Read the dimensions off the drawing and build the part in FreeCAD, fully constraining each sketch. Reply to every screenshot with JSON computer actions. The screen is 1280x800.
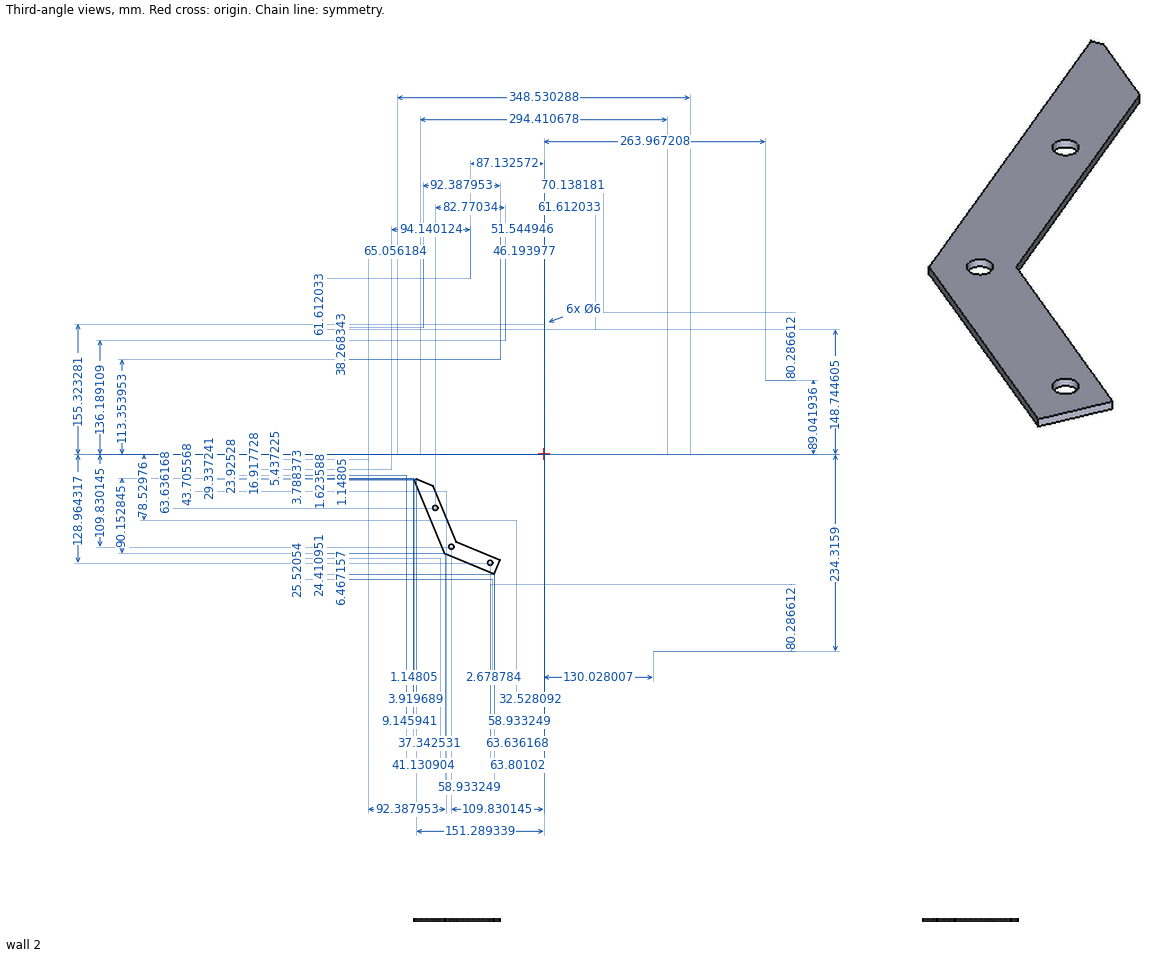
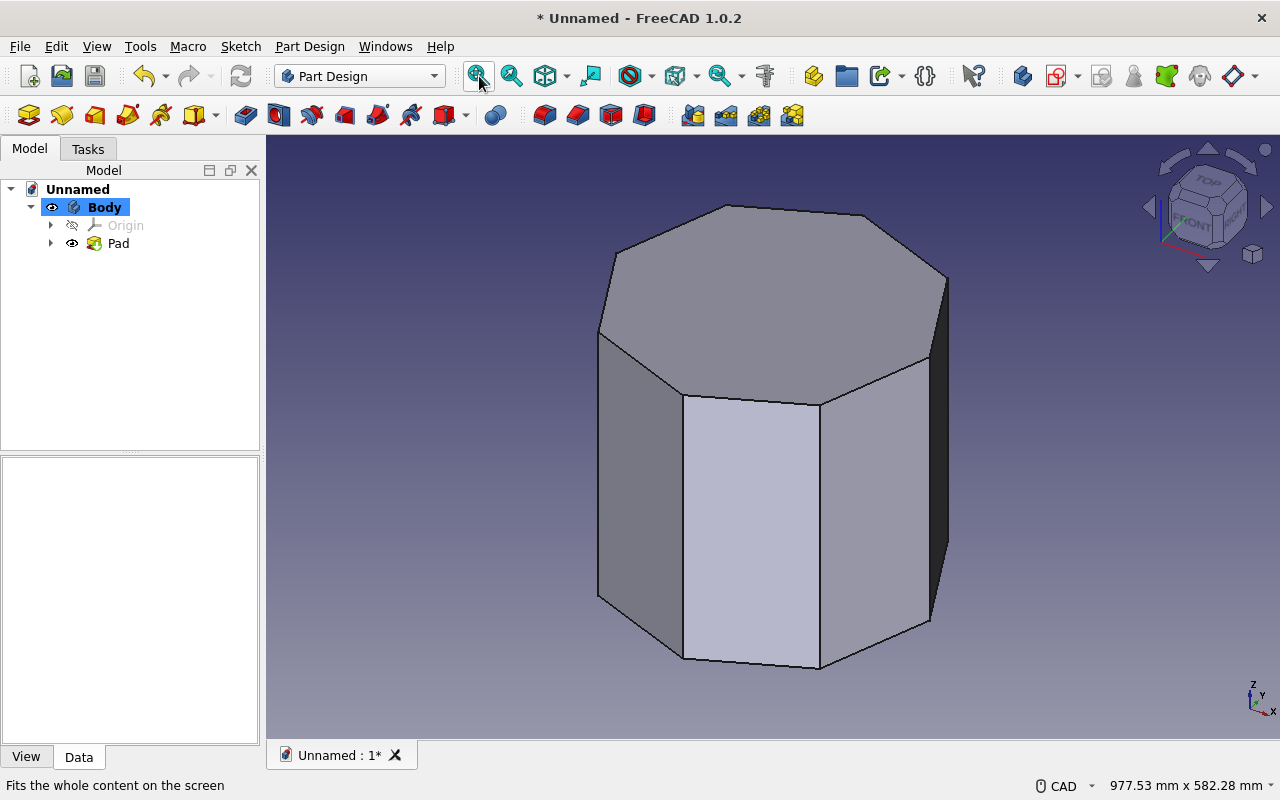
{"action": "key", "text": "0"}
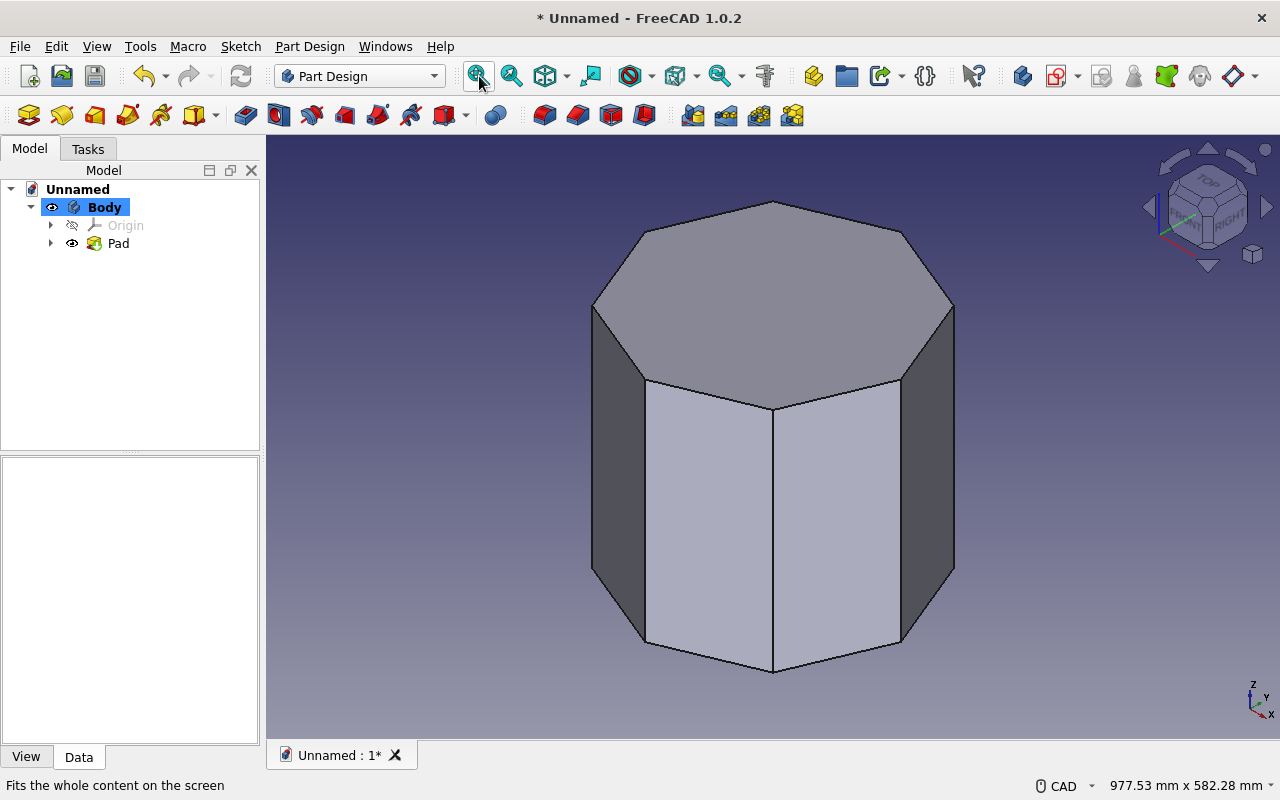
{"action": "key", "text": "2"}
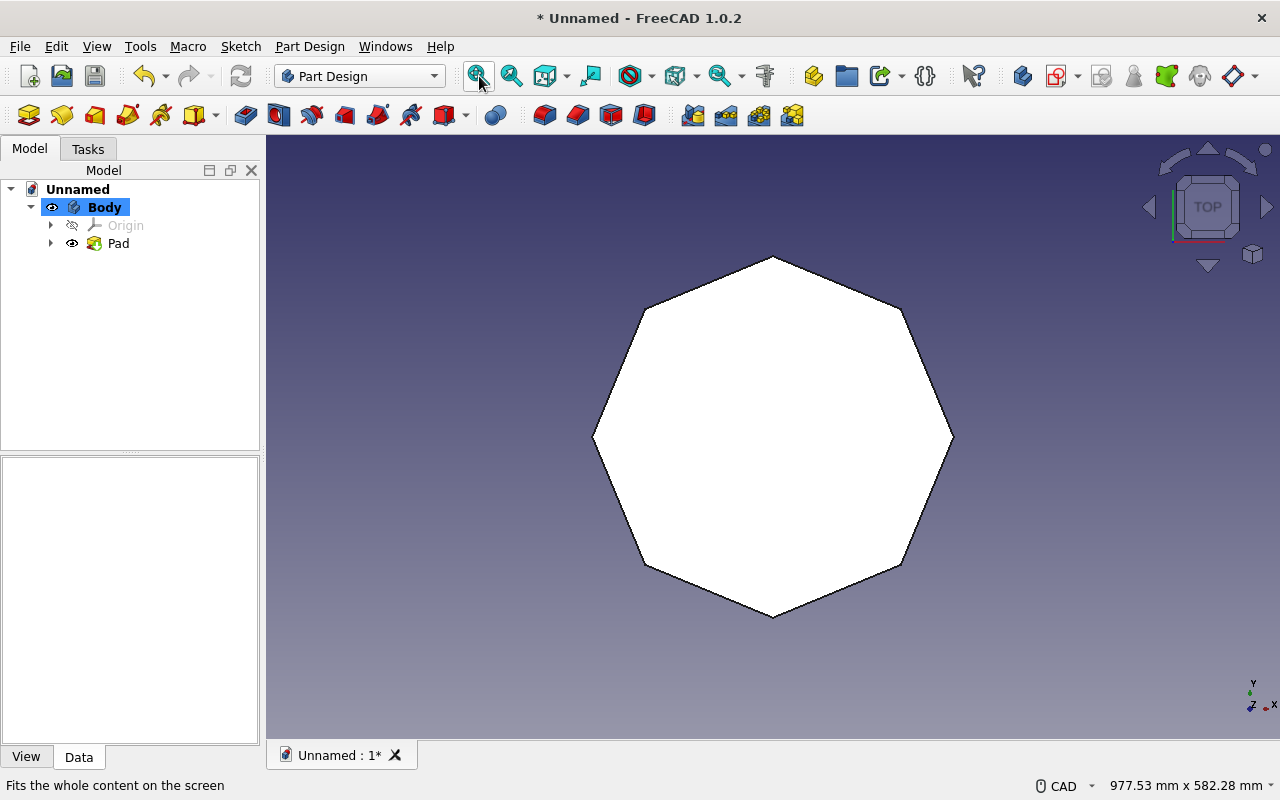
{"action": "key", "text": "1"}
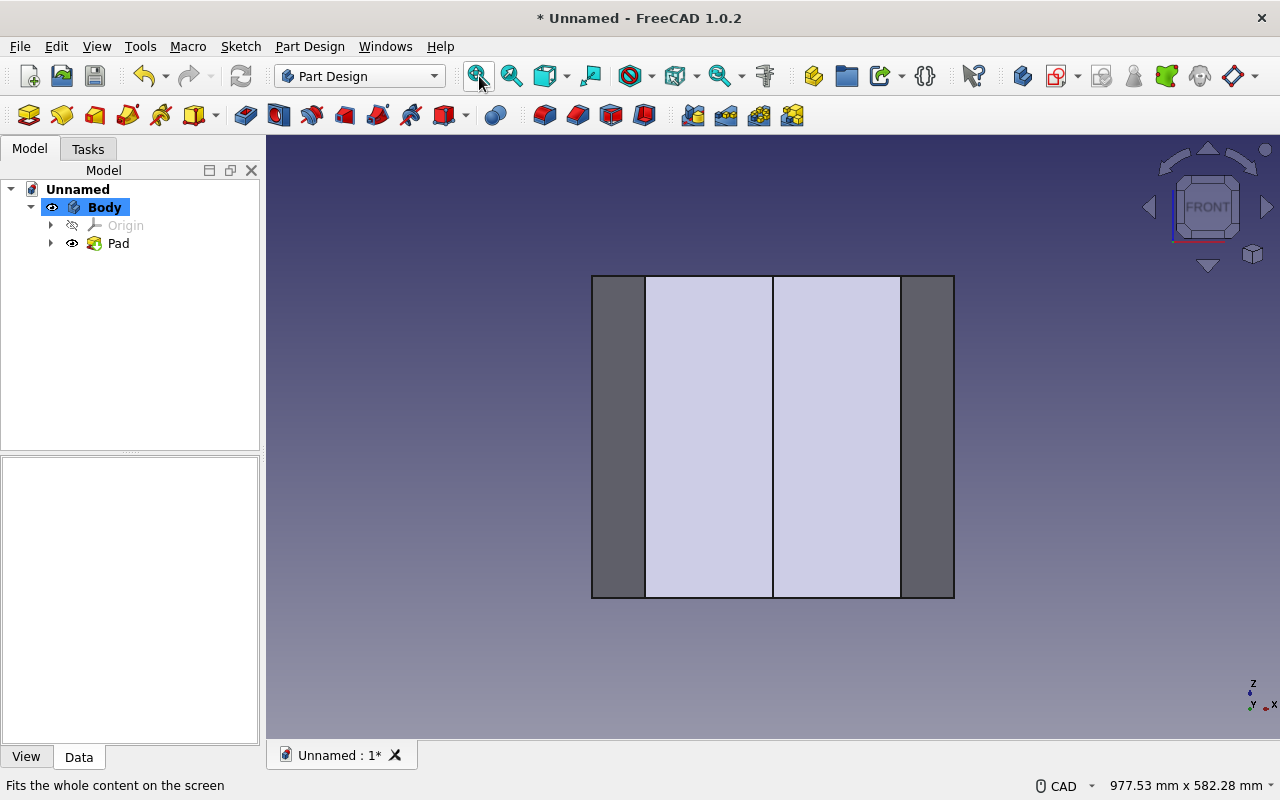
{"action": "key", "text": "3"}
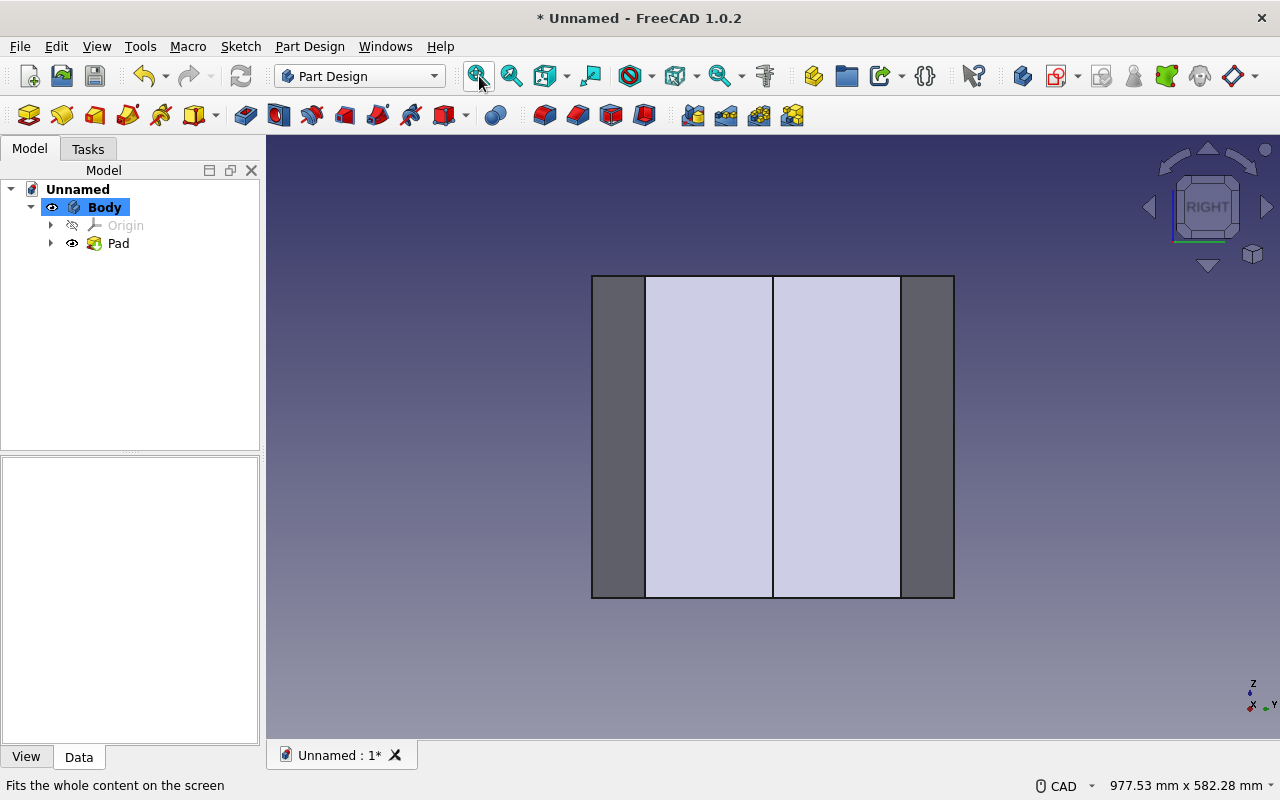
{"action": "key", "text": "5"}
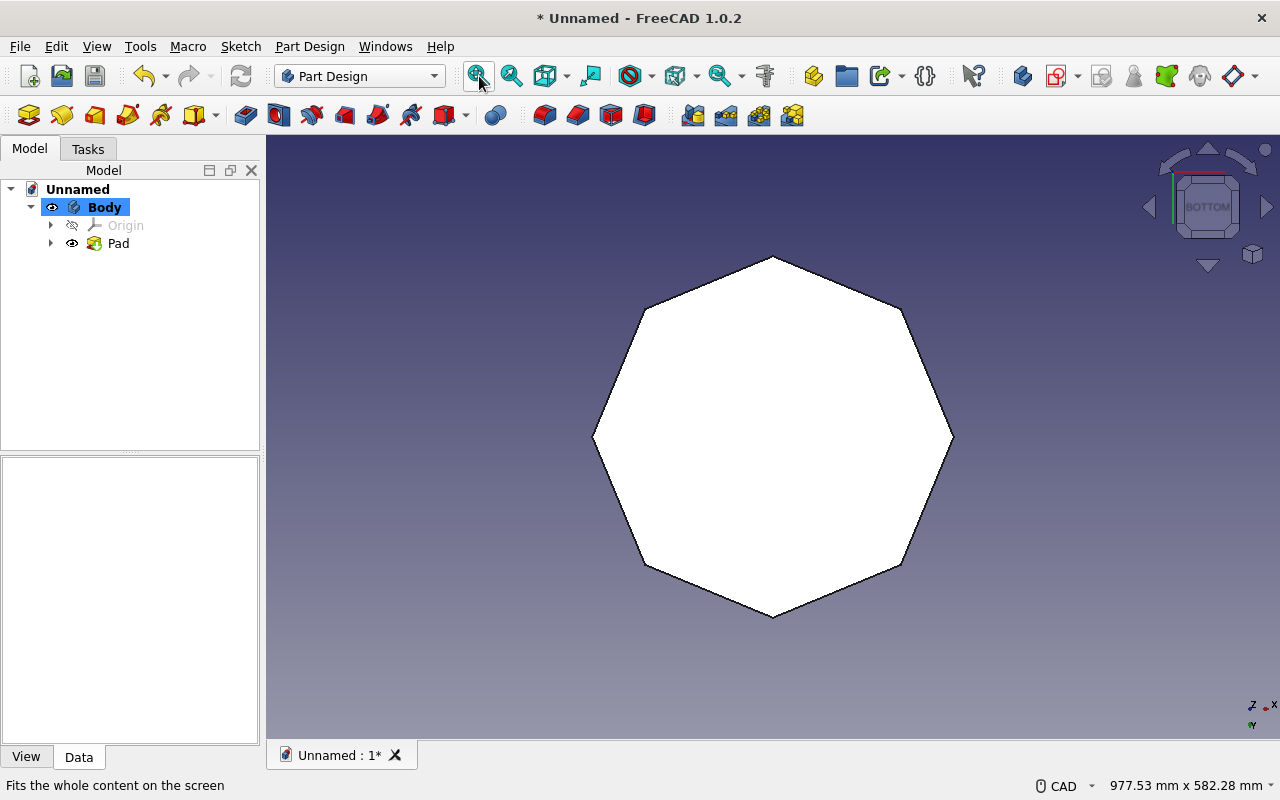
{"action": "left_click", "coordinate": [773, 436]}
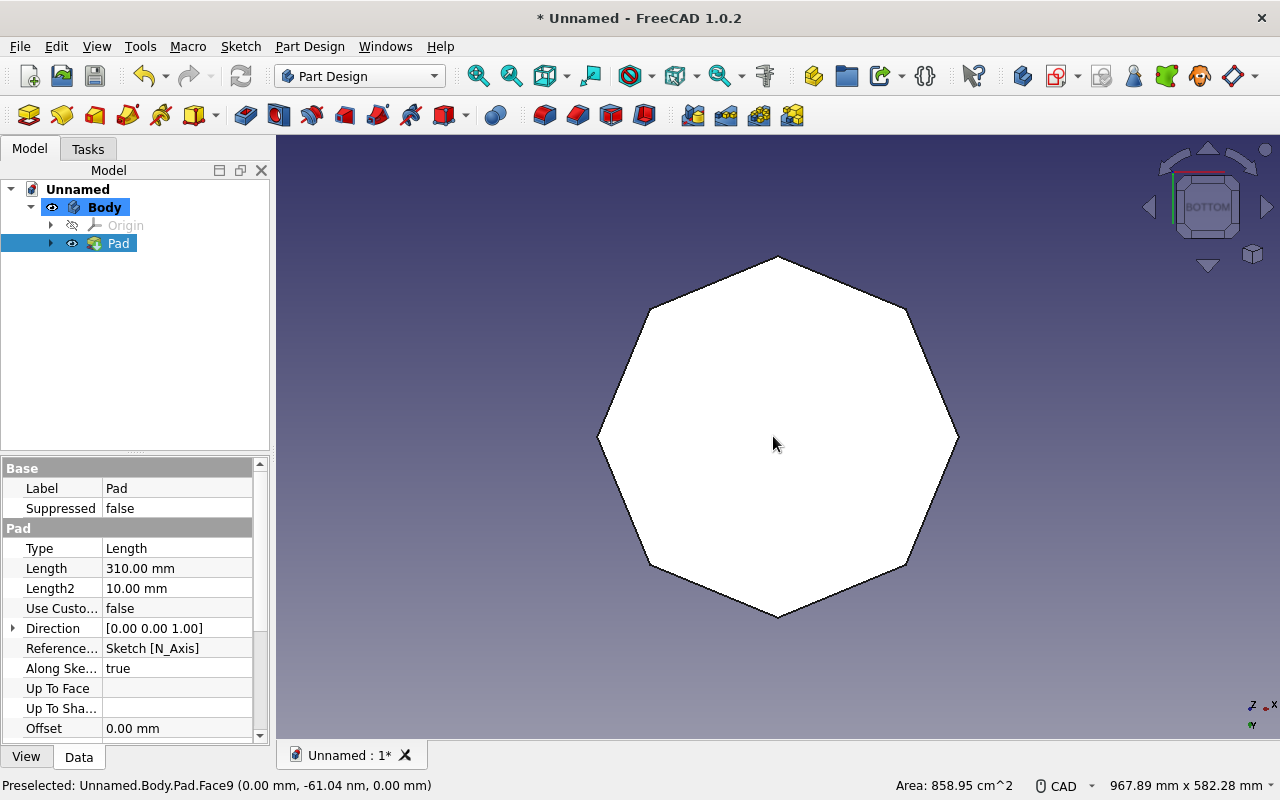
{"action": "left_click", "coordinate": [644, 116]}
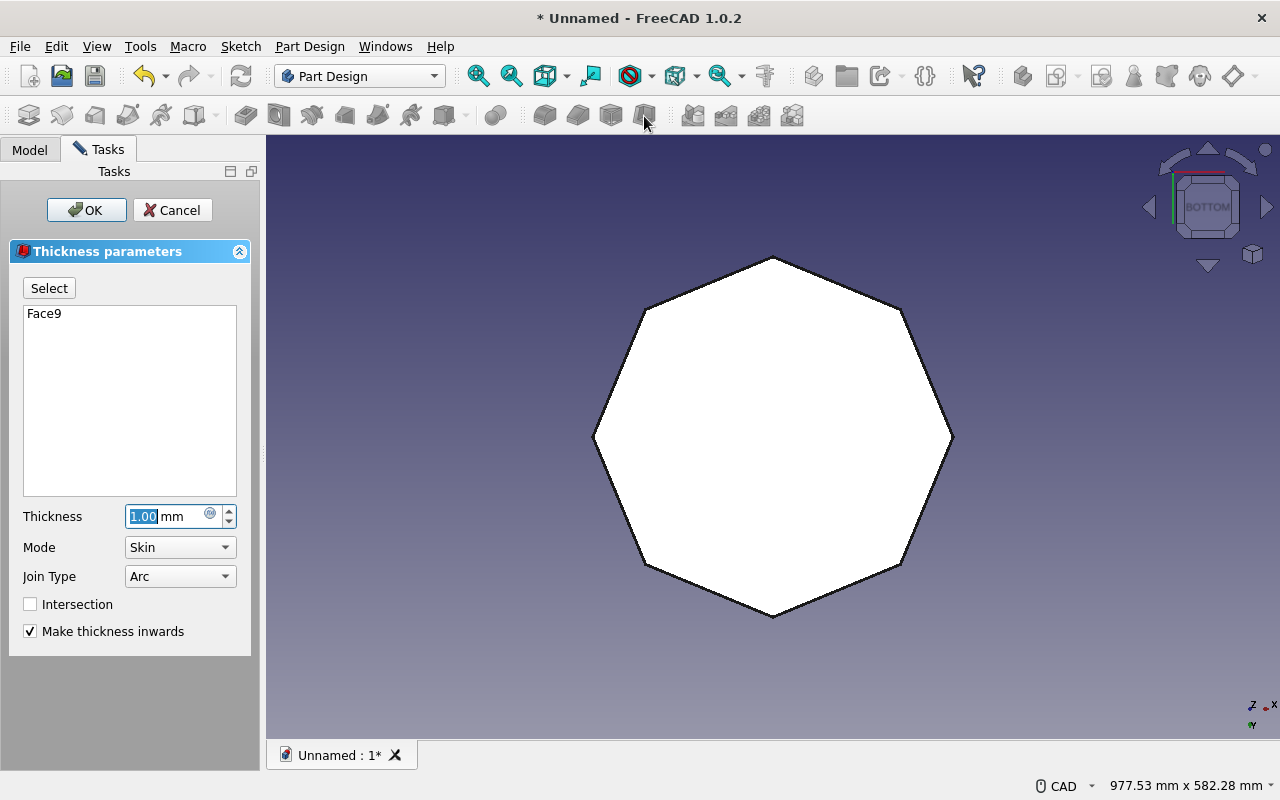
{"action": "type", "text": "2"}
{"action": "key", "text": "Tab"}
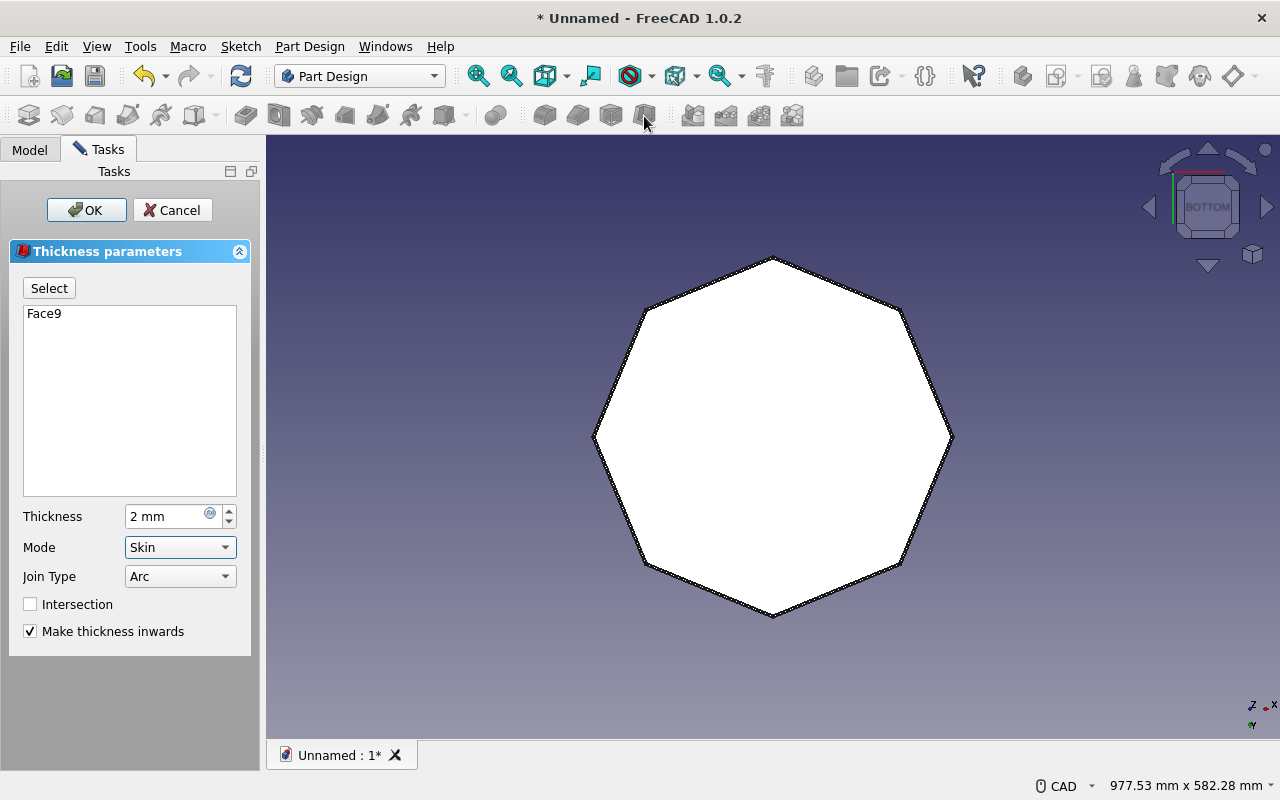
{"action": "left_click", "coordinate": [181, 576]}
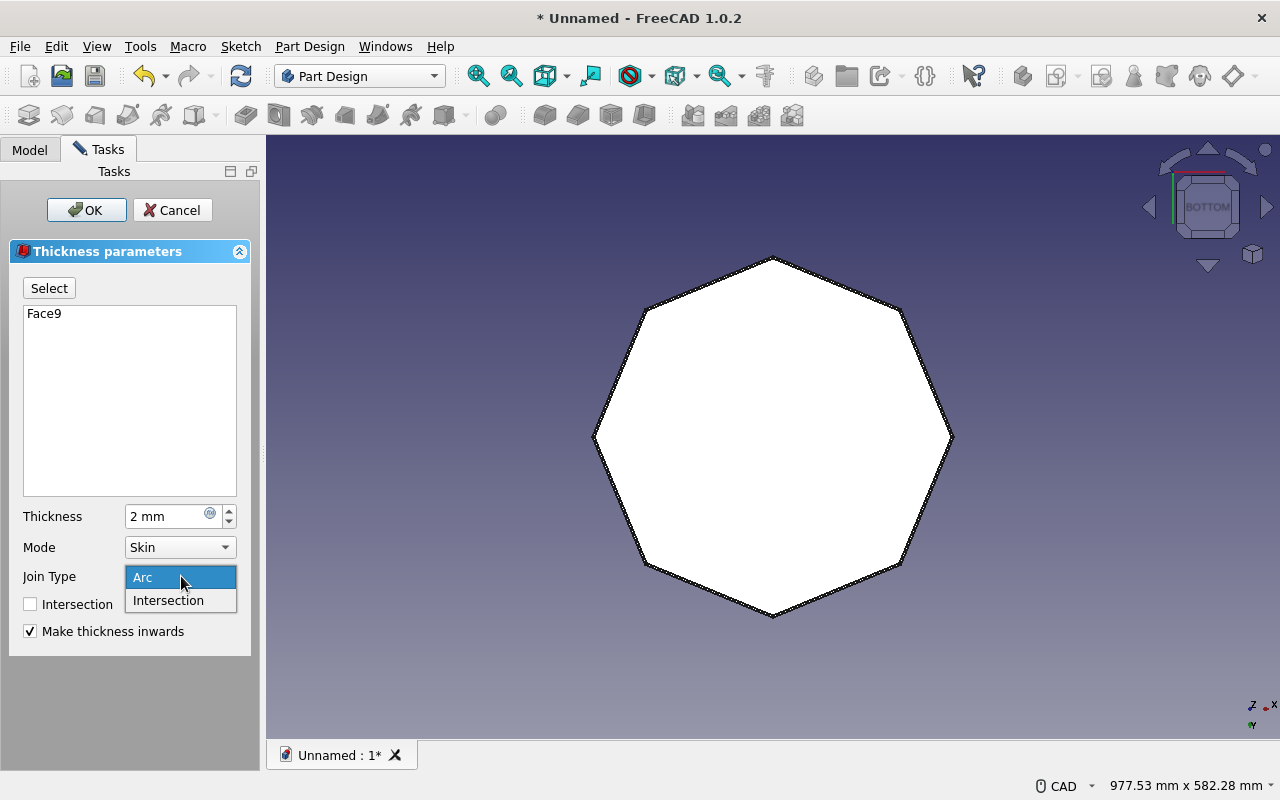
{"action": "left_click", "coordinate": [179, 600]}